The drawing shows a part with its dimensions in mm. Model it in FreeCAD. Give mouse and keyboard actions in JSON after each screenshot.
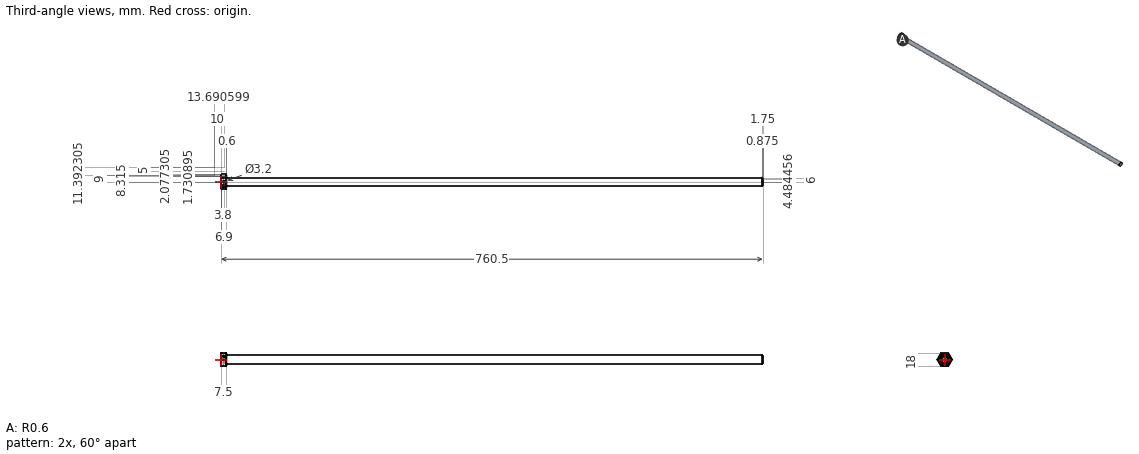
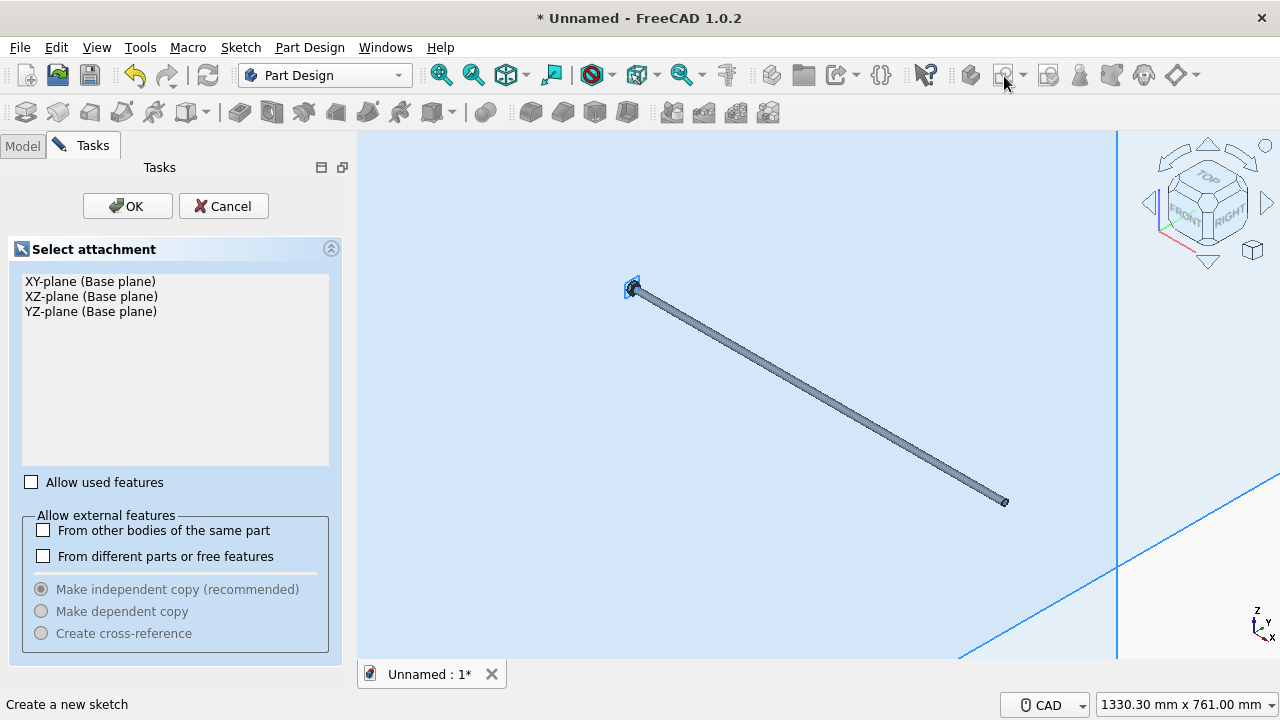
{"action": "left_click", "coordinate": [82, 282]}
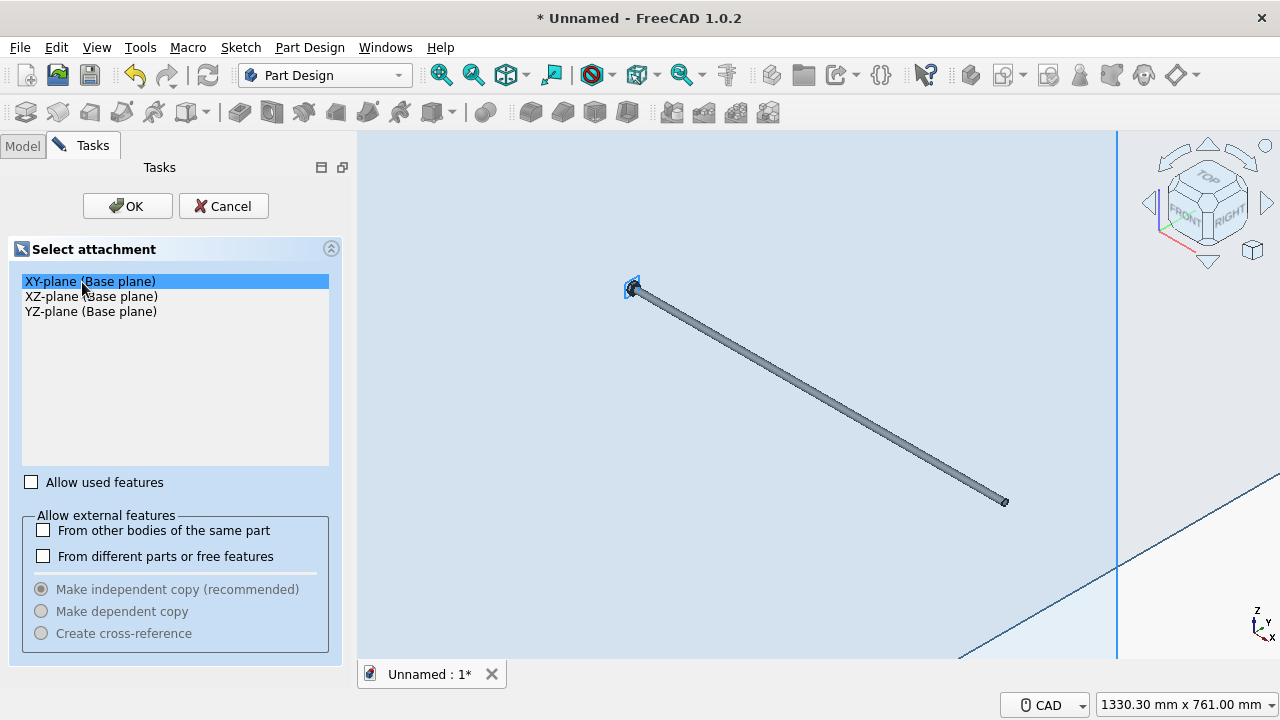
{"action": "left_click", "coordinate": [128, 206]}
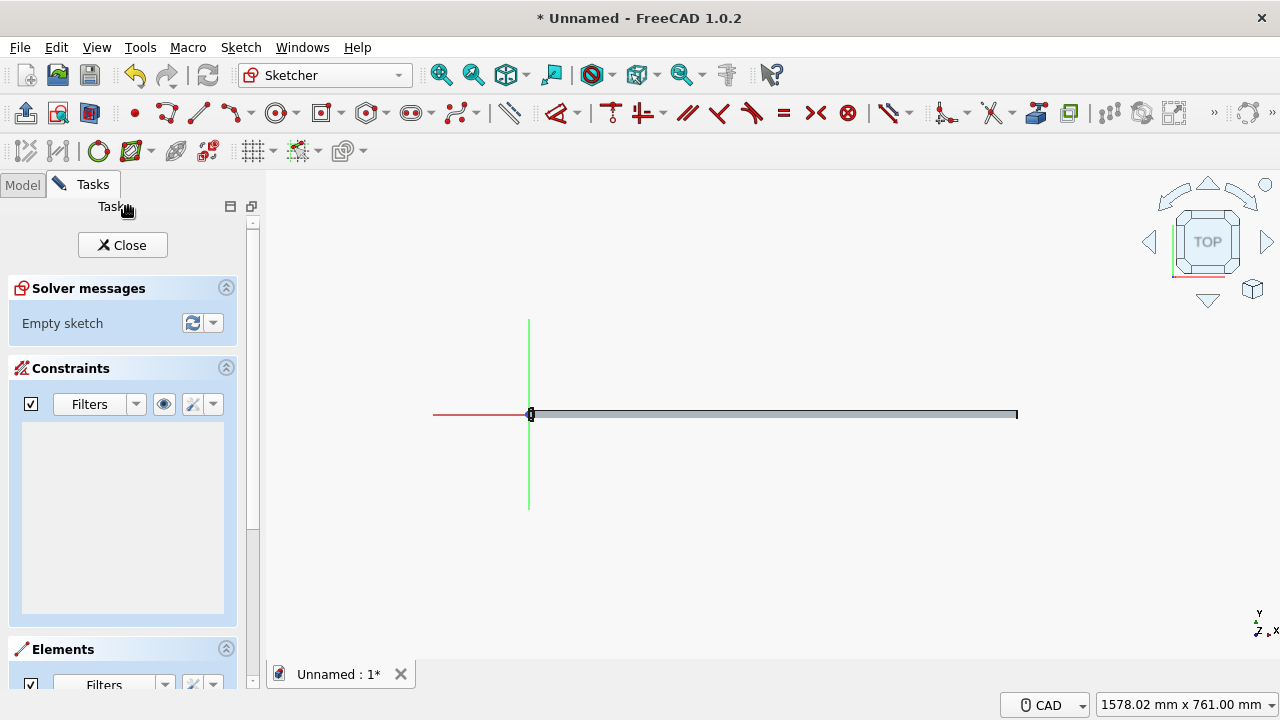
{"action": "key", "text": "q s"}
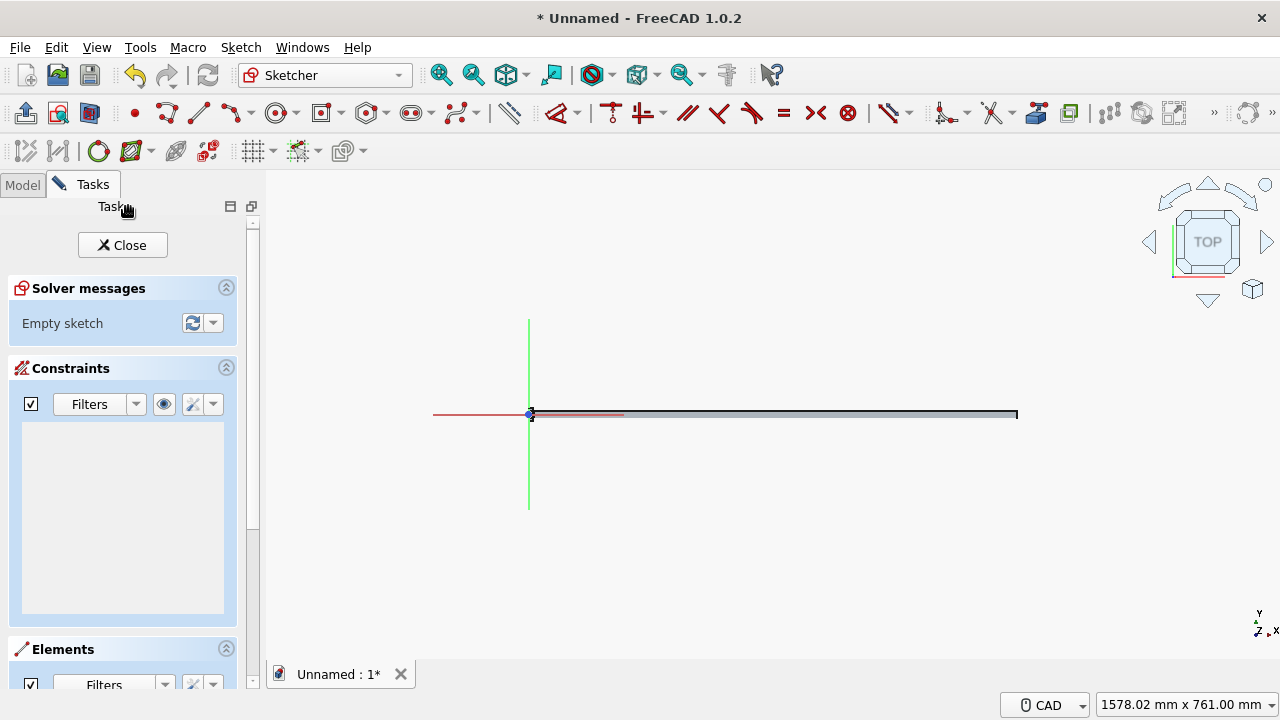
{"action": "scroll", "coordinate": [1034, 411], "scroll_direction": "up", "scroll_amount": 15}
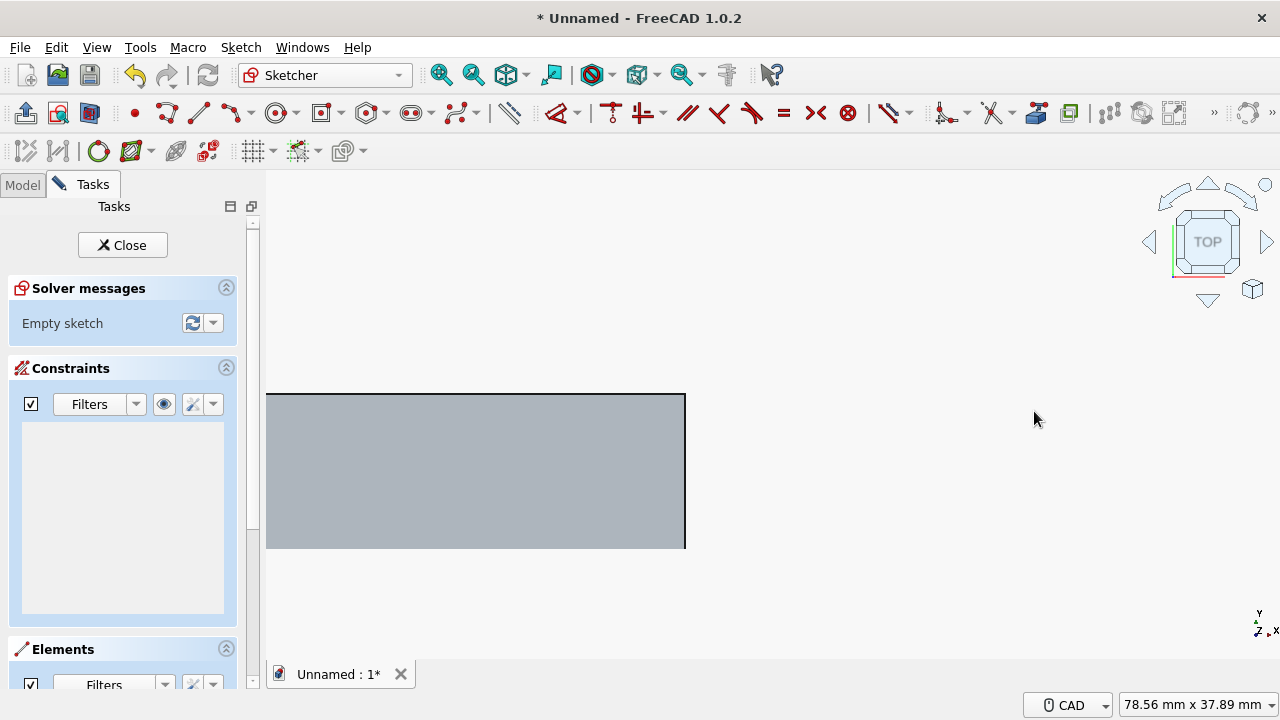
{"action": "scroll", "coordinate": [684, 404], "scroll_direction": "up", "scroll_amount": 14}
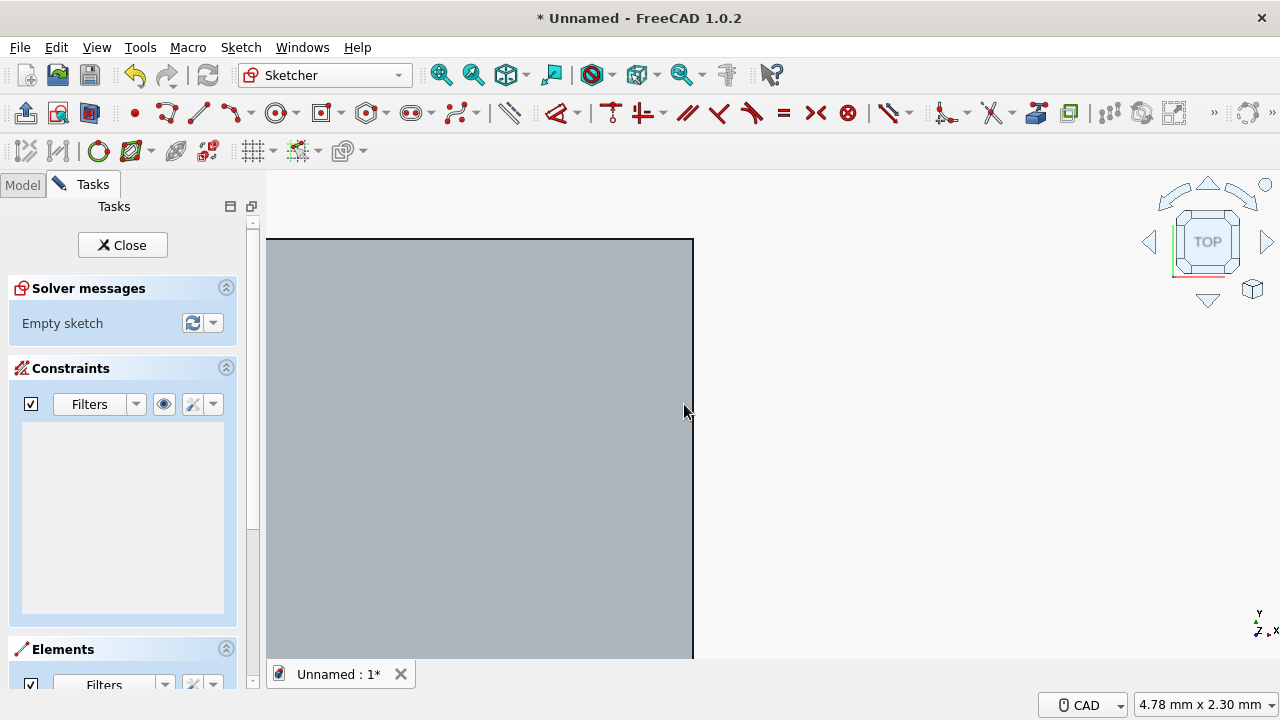
{"action": "key", "text": "g m"}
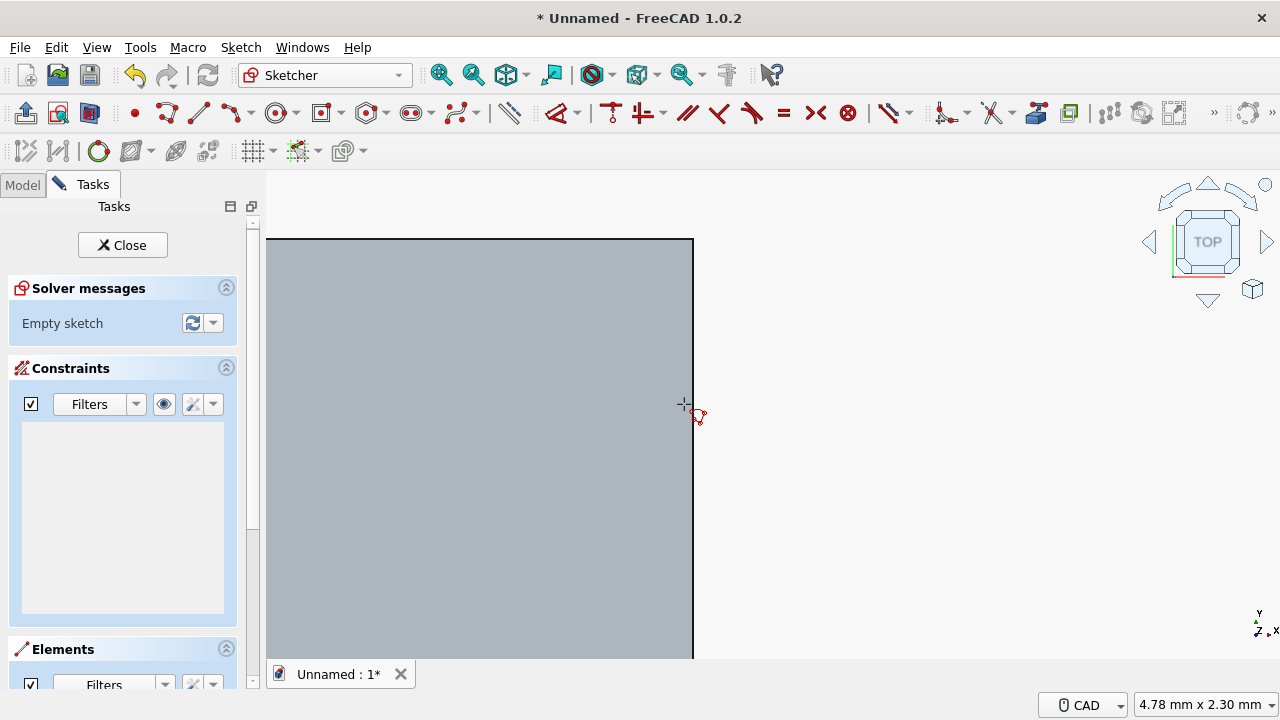
{"action": "left_click", "coordinate": [507, 239]}
{"action": "left_click", "coordinate": [693, 561]}
{"action": "left_click", "coordinate": [878, 239]}
{"action": "left_click", "coordinate": [507, 240]}
{"action": "key", "text": "Escape"}
{"action": "key", "text": "Escape"}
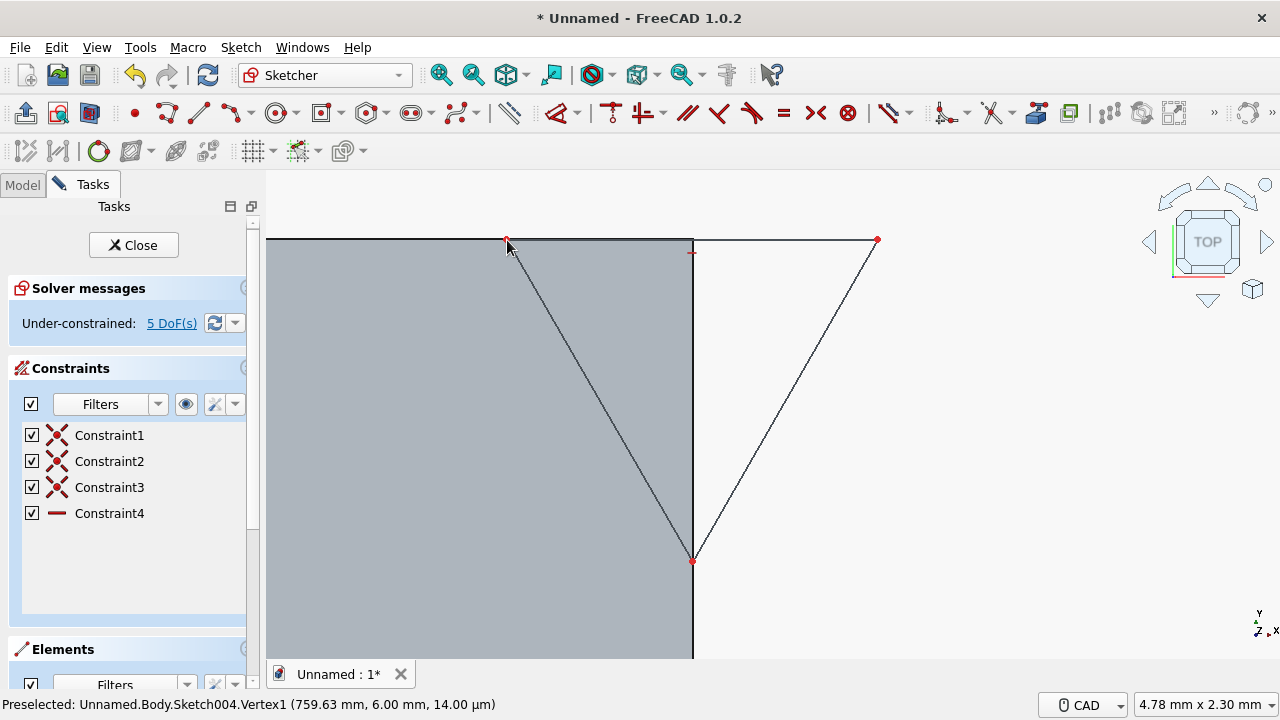
{"action": "key", "text": "d"}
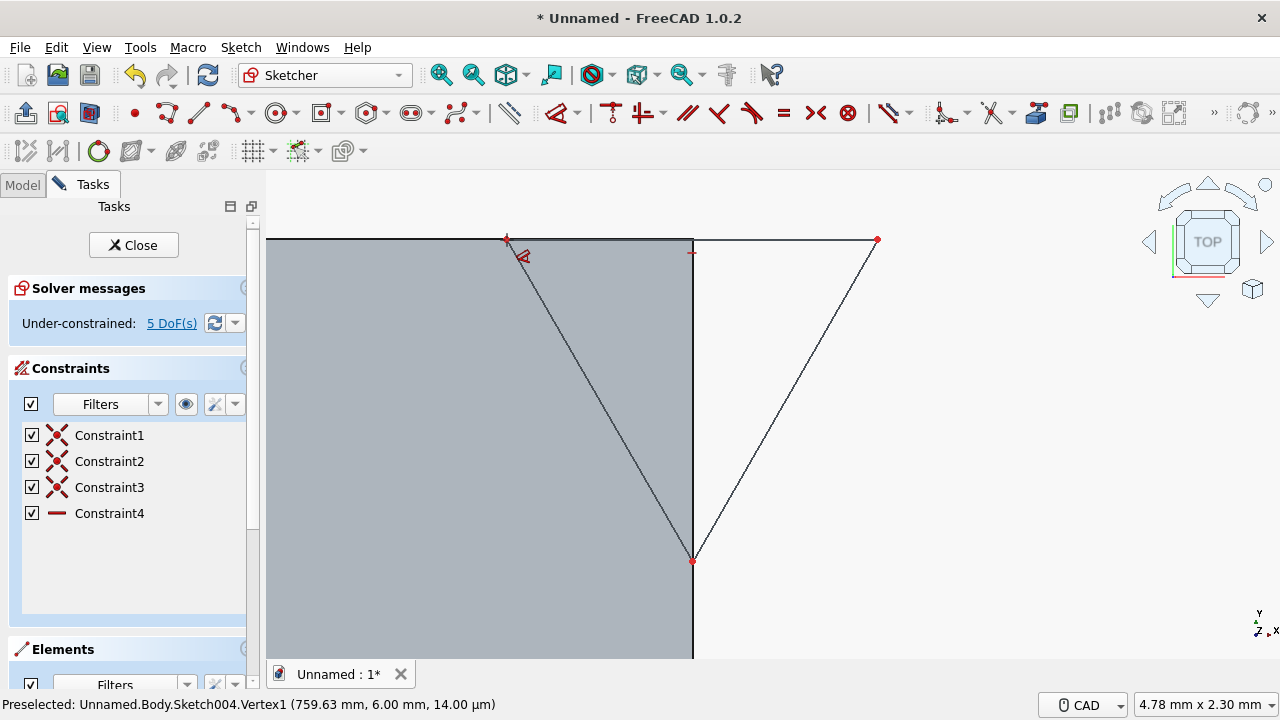
{"action": "left_click", "coordinate": [507, 240]}
{"action": "left_click", "coordinate": [541, 435]}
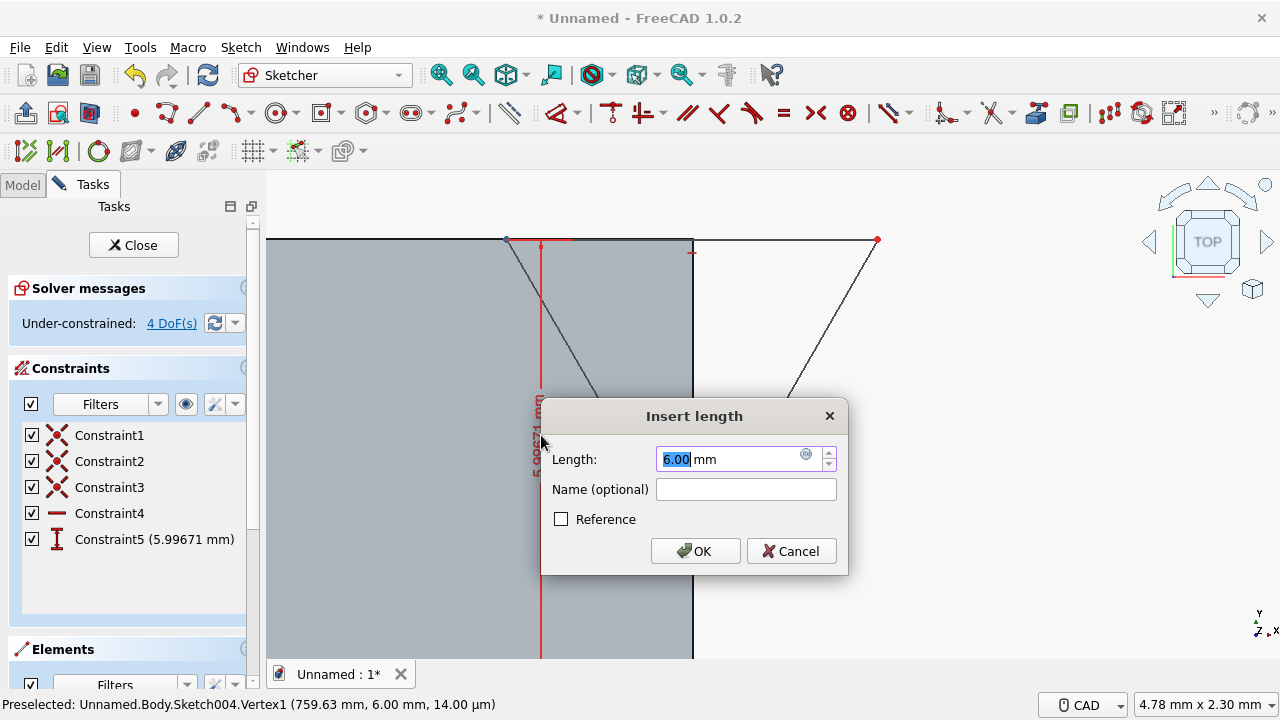
{"action": "type", "text": "6"}
{"action": "key", "text": "Return"}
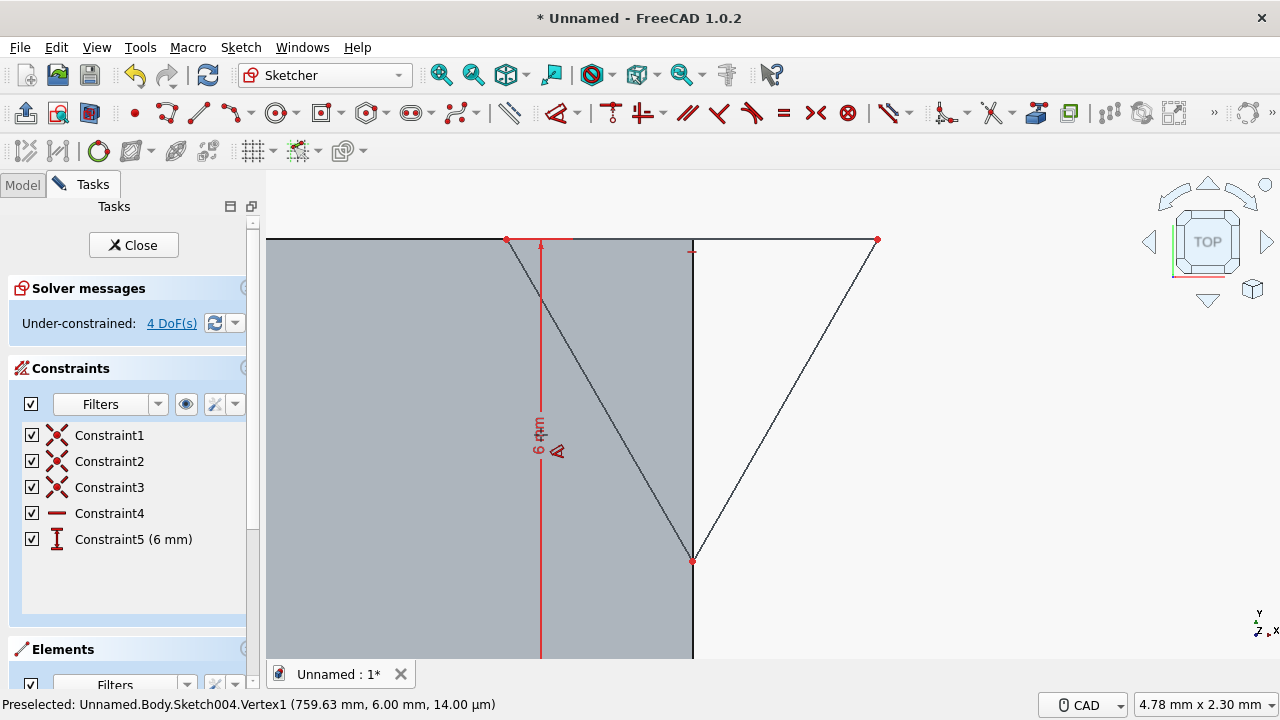
{"action": "left_click", "coordinate": [767, 239]}
{"action": "left_click", "coordinate": [692, 205]}